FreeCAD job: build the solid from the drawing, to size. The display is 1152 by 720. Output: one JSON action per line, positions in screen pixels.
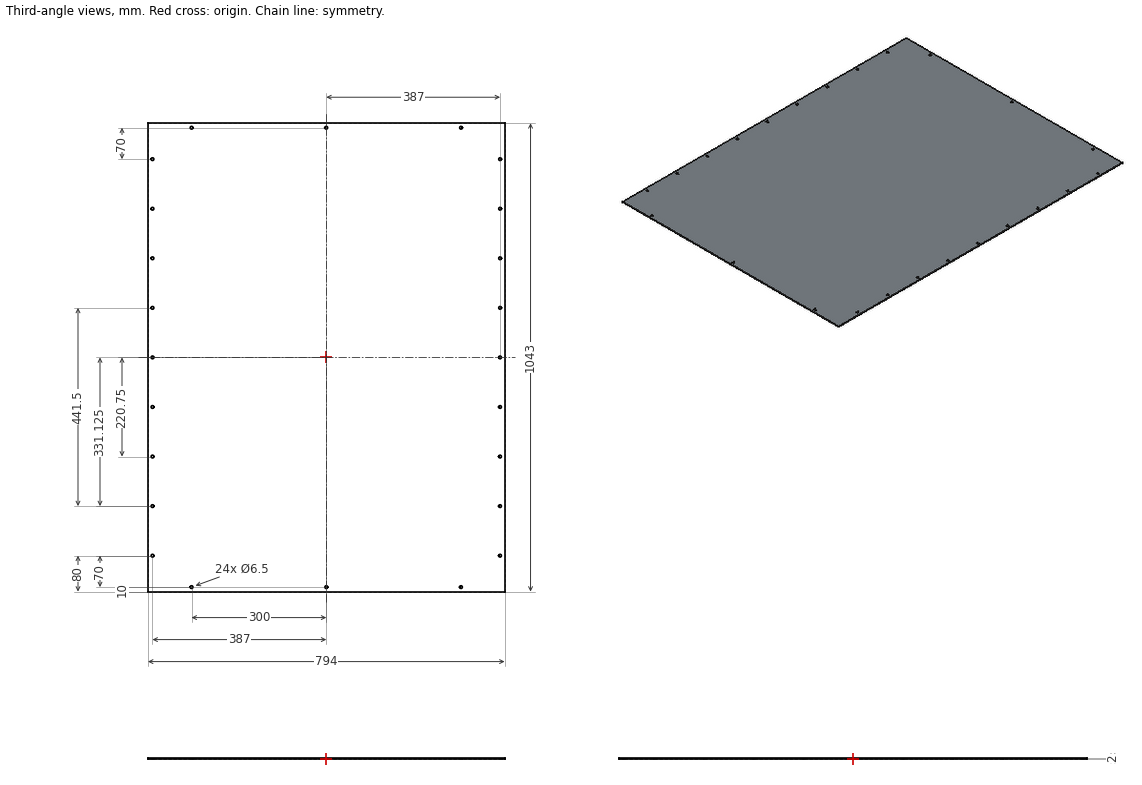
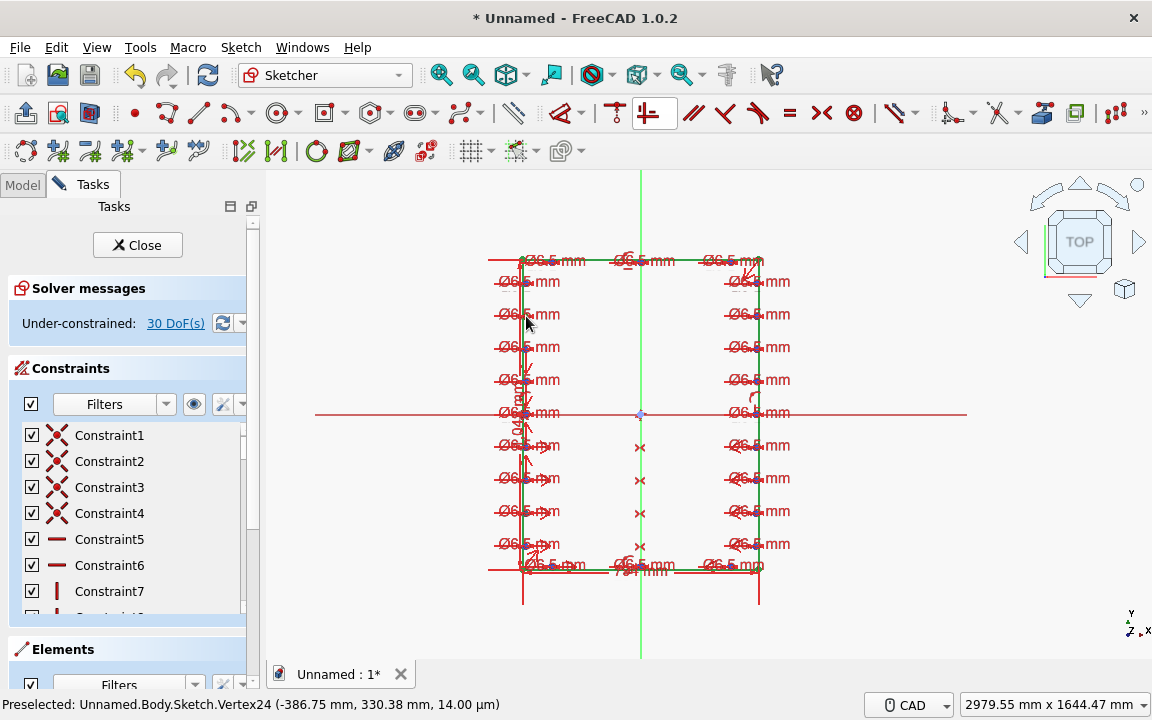
{"action": "left_click", "coordinate": [344, 415]}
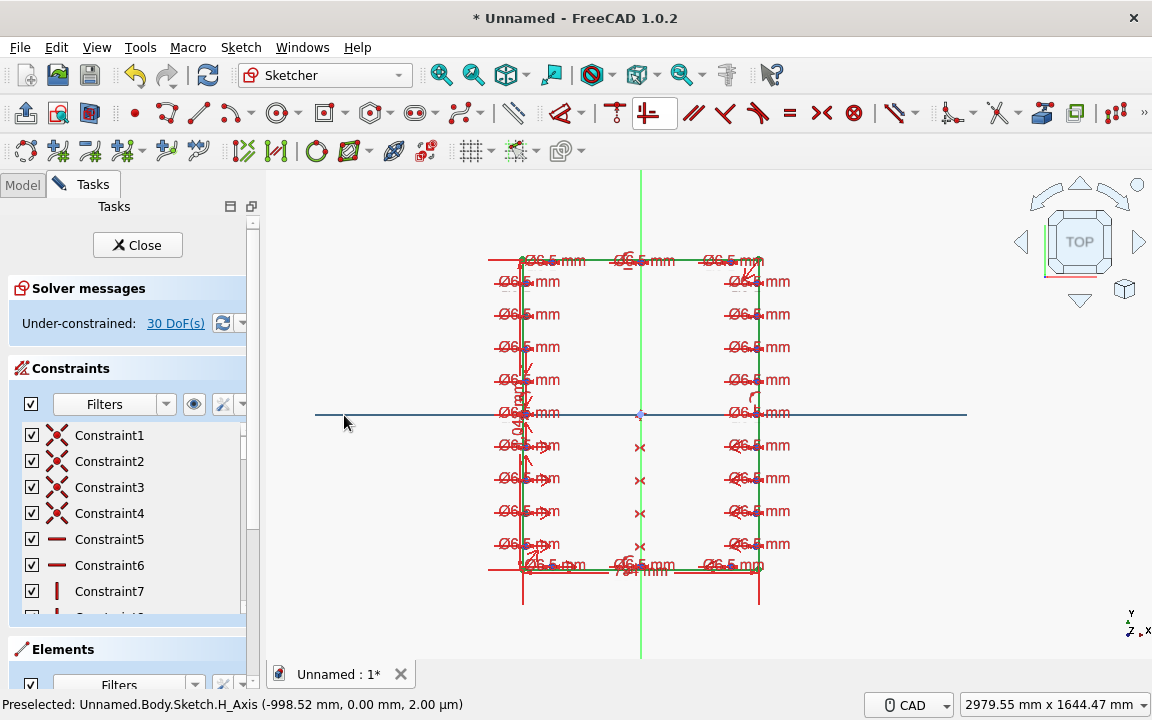
{"action": "left_click", "coordinate": [822, 114]}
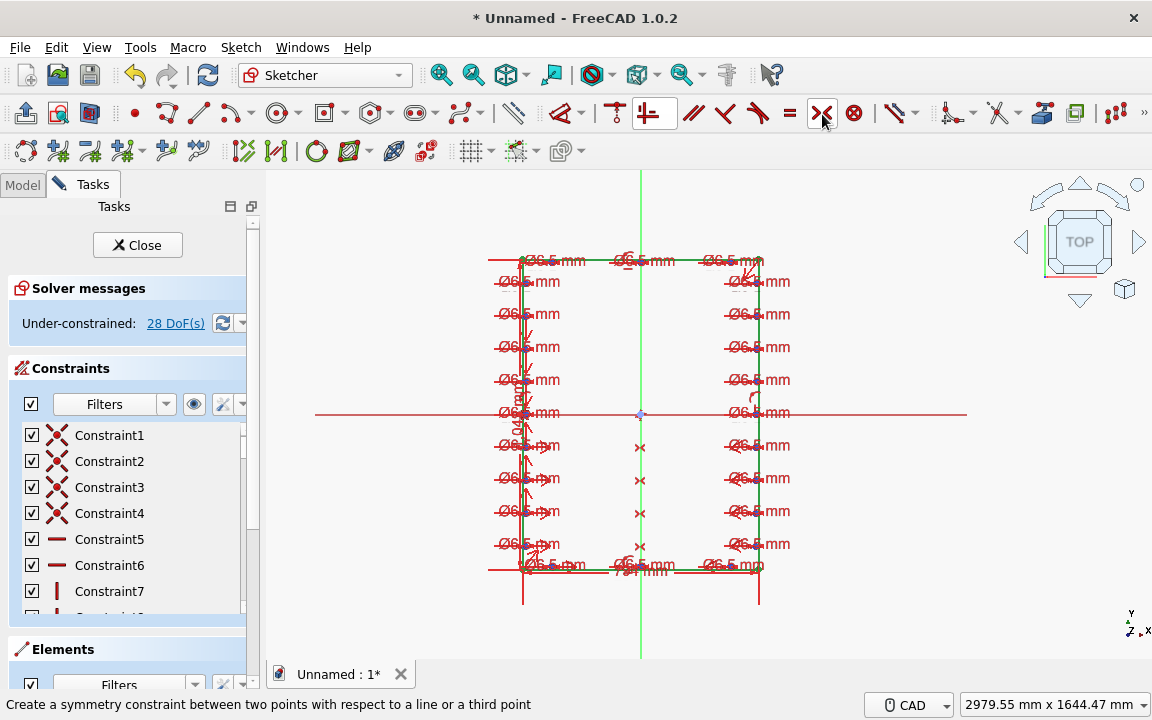
{"action": "left_click", "coordinate": [526, 546]}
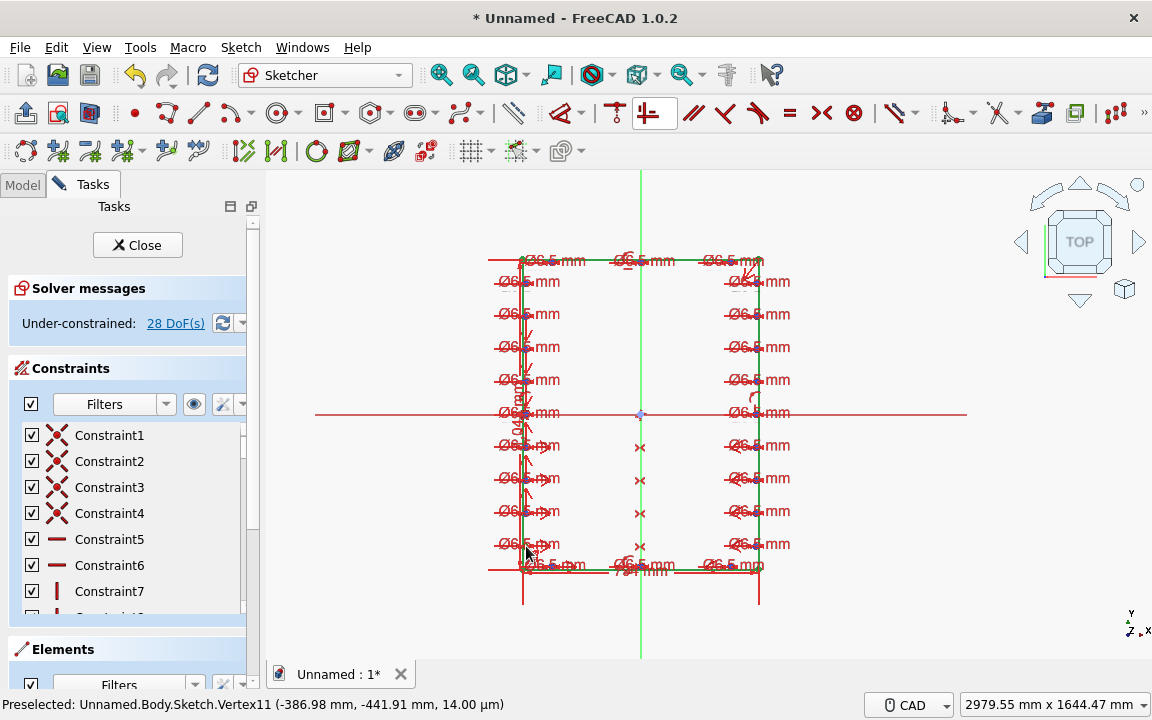
{"action": "left_click", "coordinate": [526, 284]}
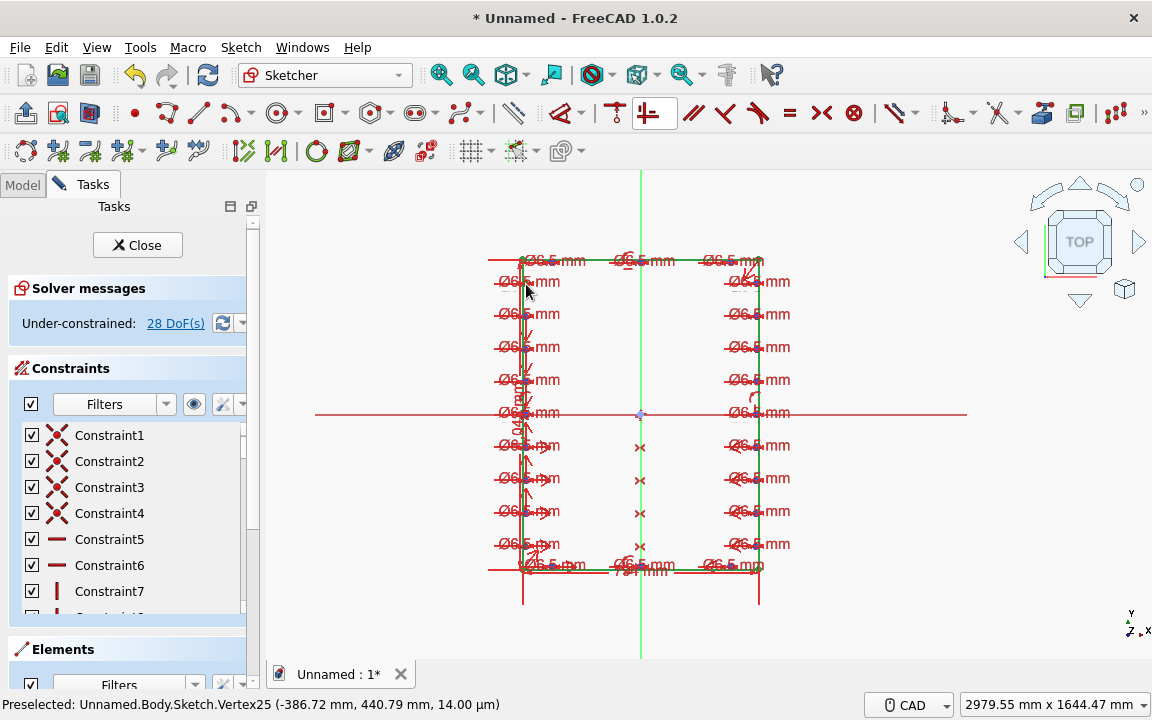
{"action": "left_click", "coordinate": [344, 415]}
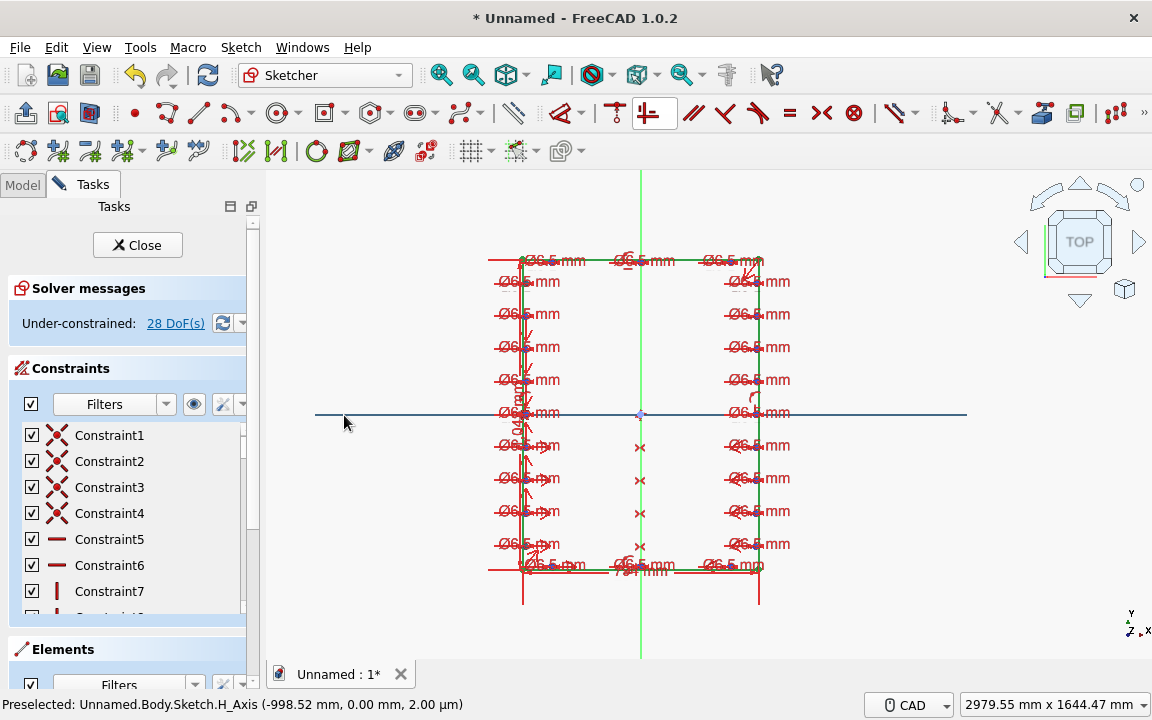
{"action": "left_click", "coordinate": [822, 114]}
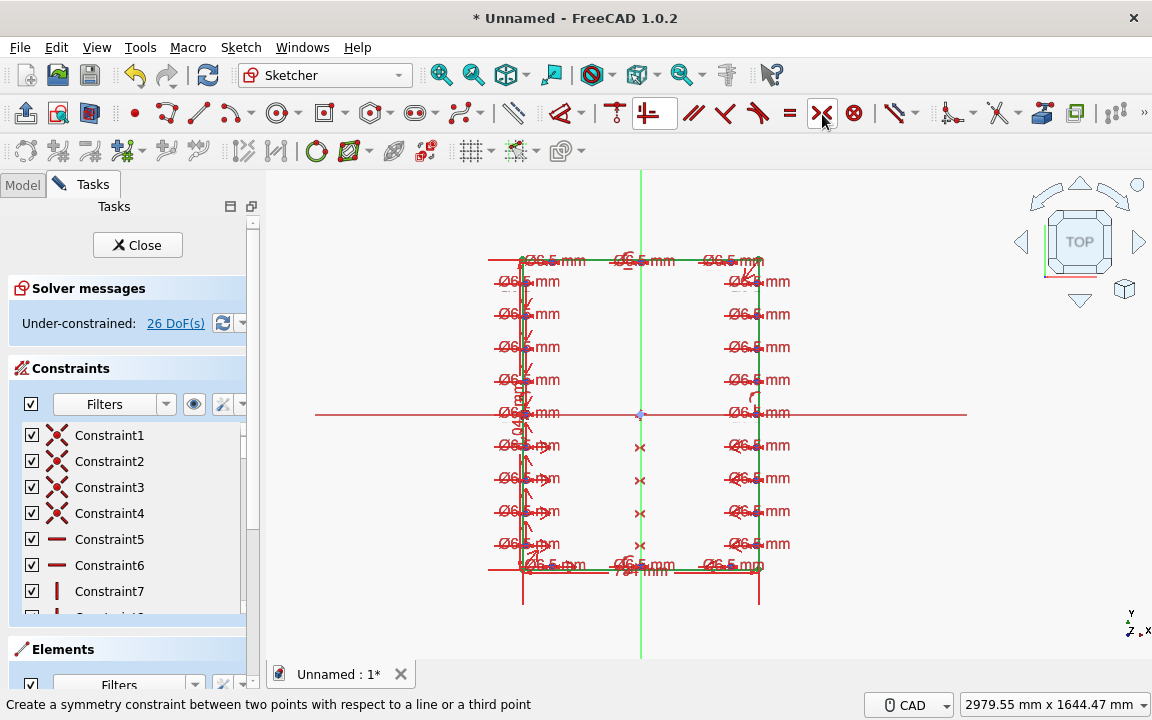
{"action": "left_click", "coordinate": [552, 567]}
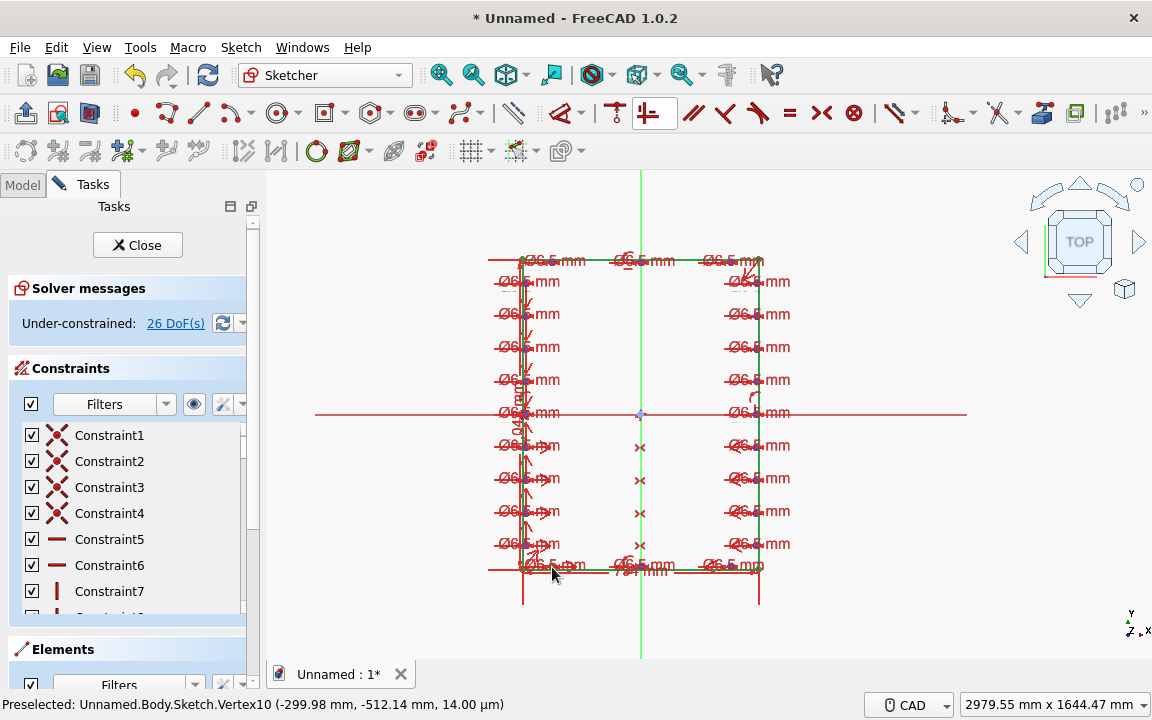
{"action": "left_click", "coordinate": [552, 263]}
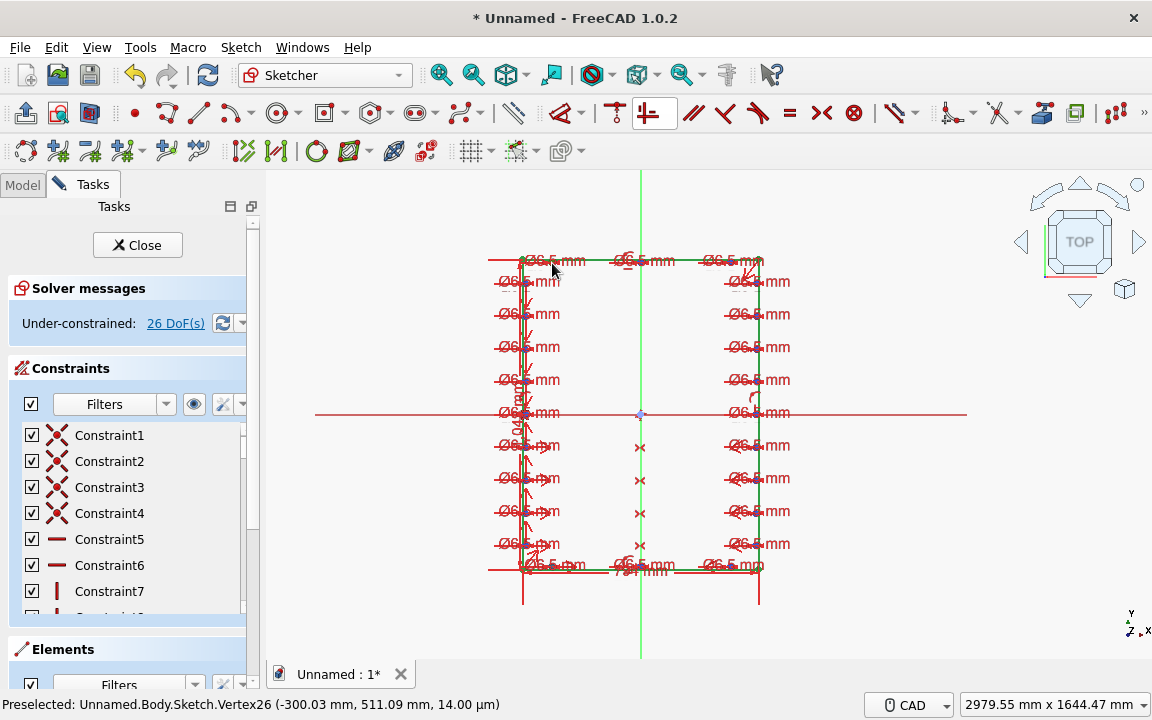
{"action": "left_click", "coordinate": [344, 415]}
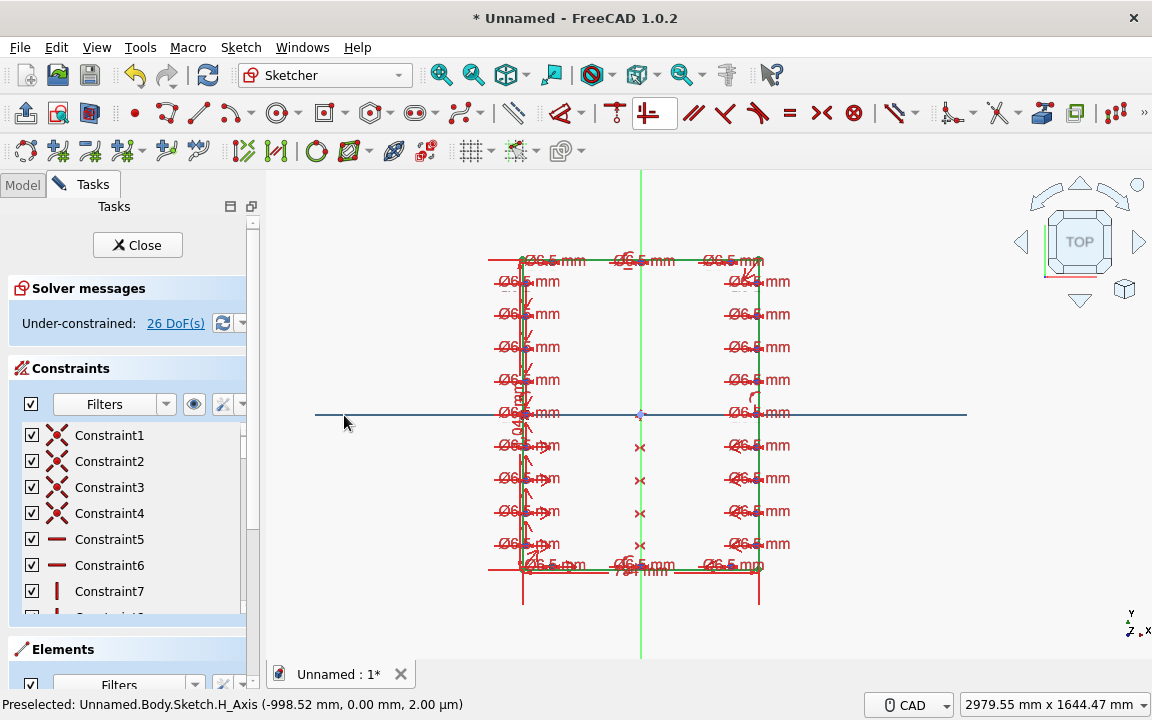
{"action": "left_click", "coordinate": [822, 114]}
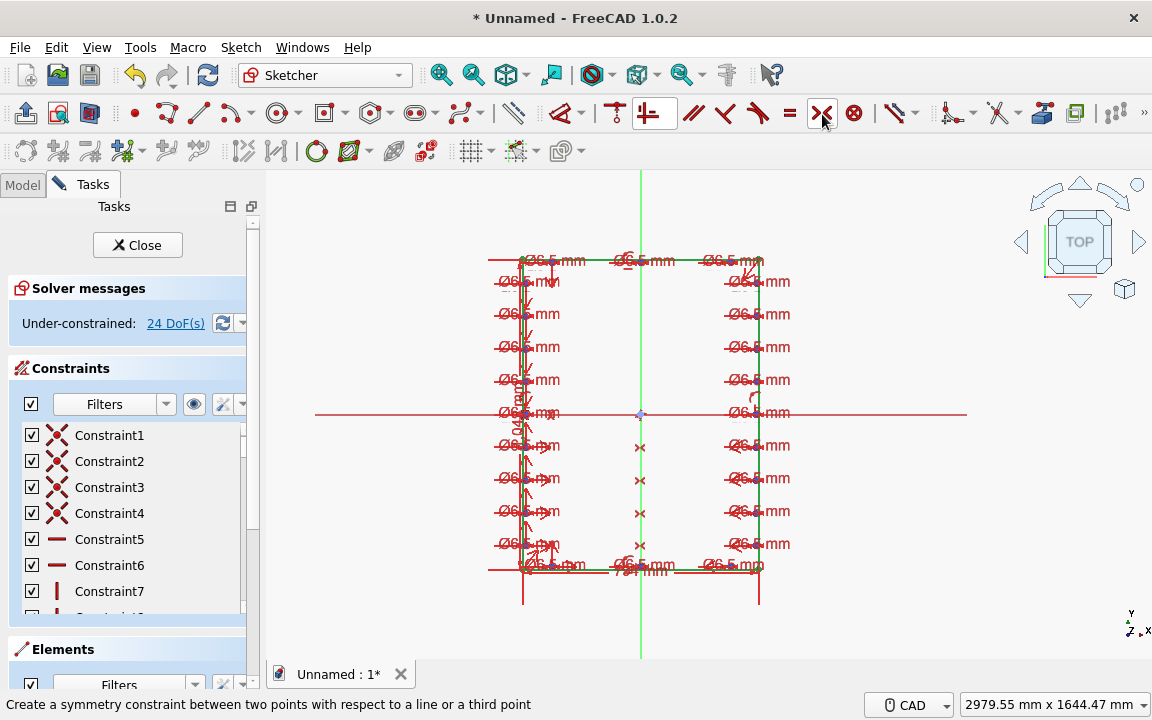
{"action": "left_click", "coordinate": [756, 447]}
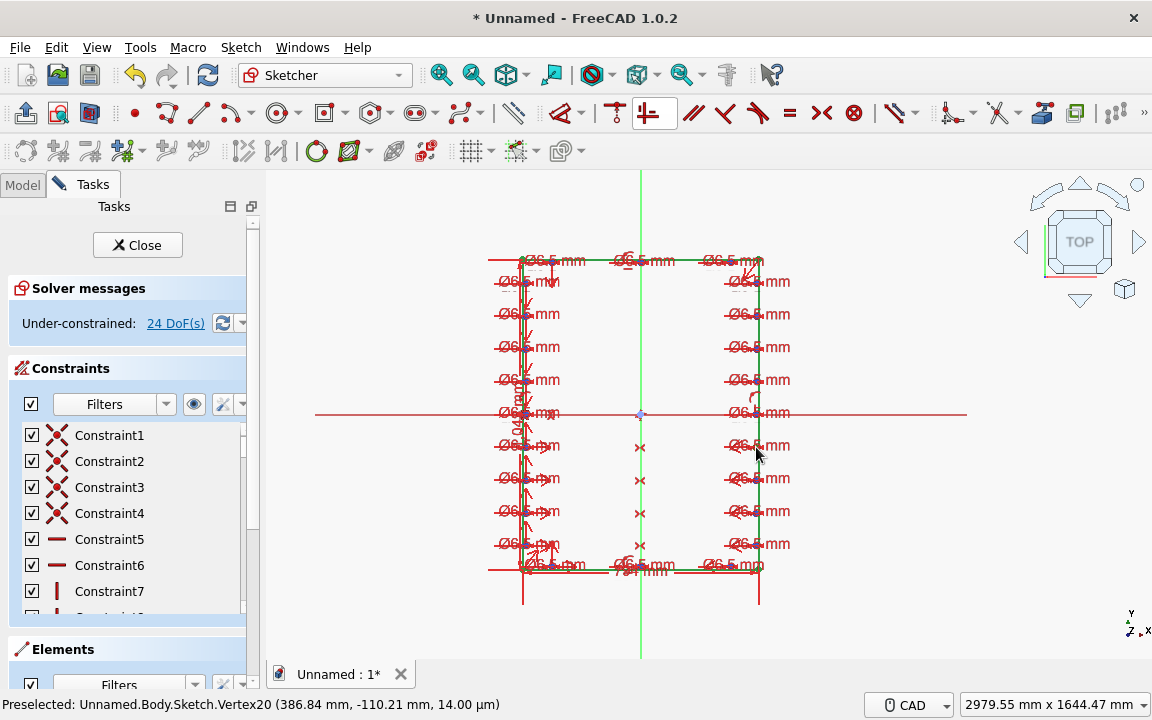
{"action": "left_click", "coordinate": [756, 382]}